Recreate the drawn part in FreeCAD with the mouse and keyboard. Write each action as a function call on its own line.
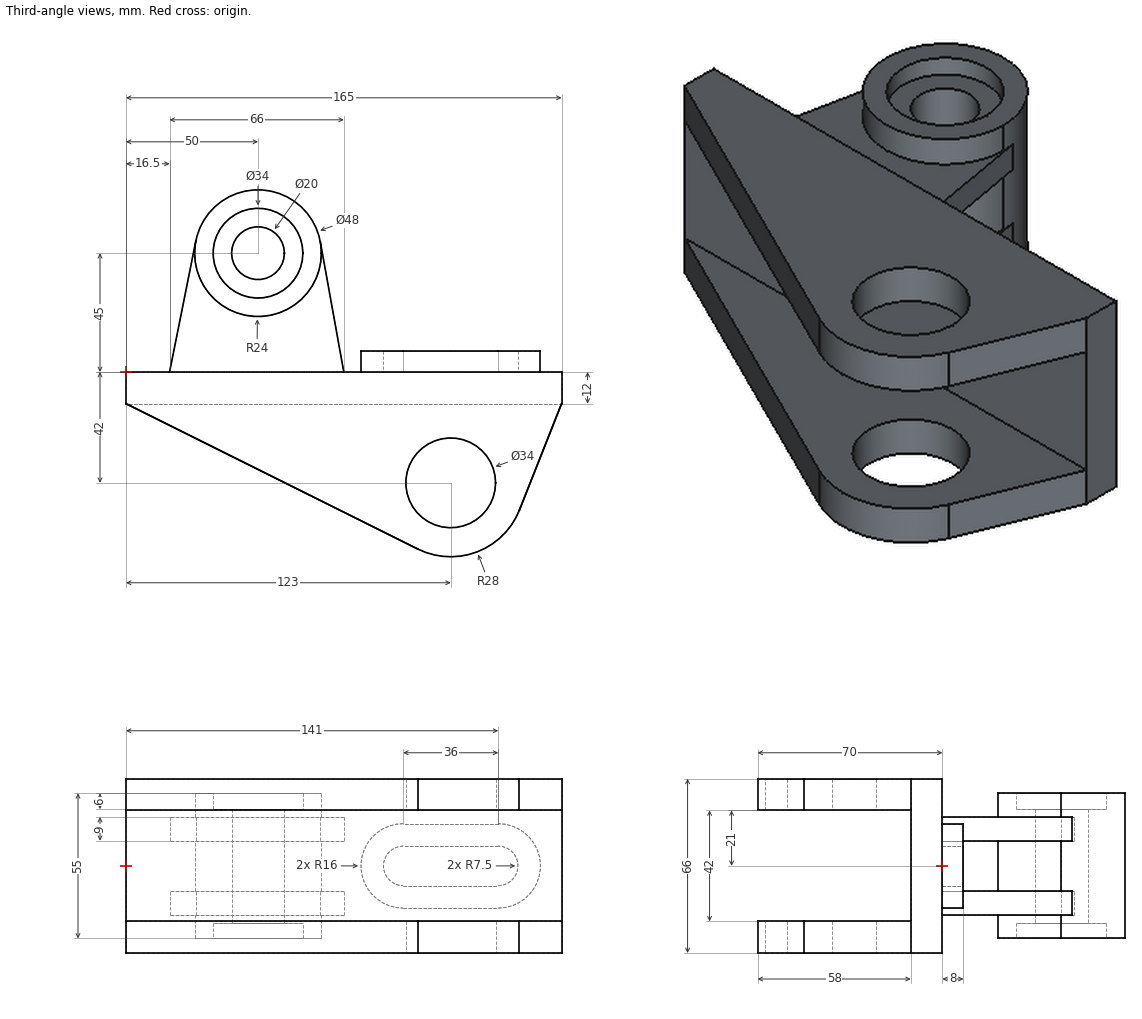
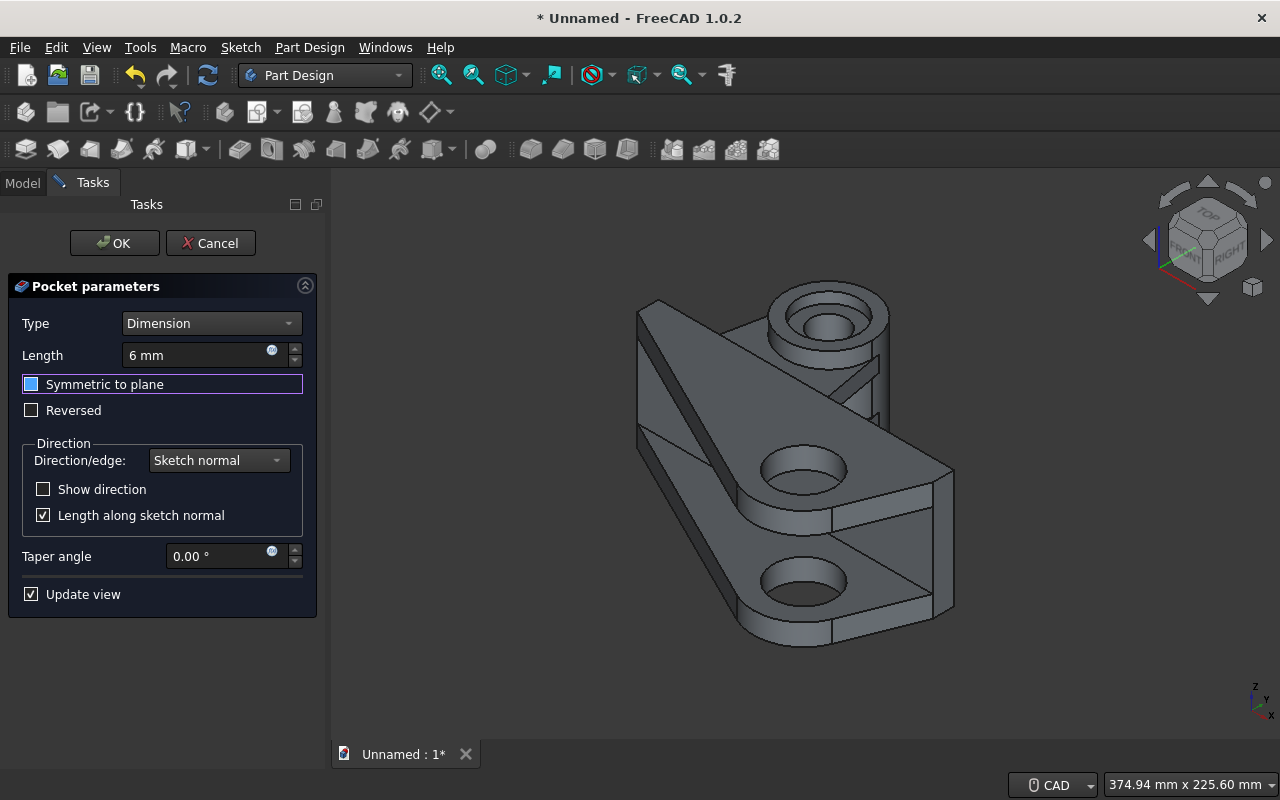
click(115, 243)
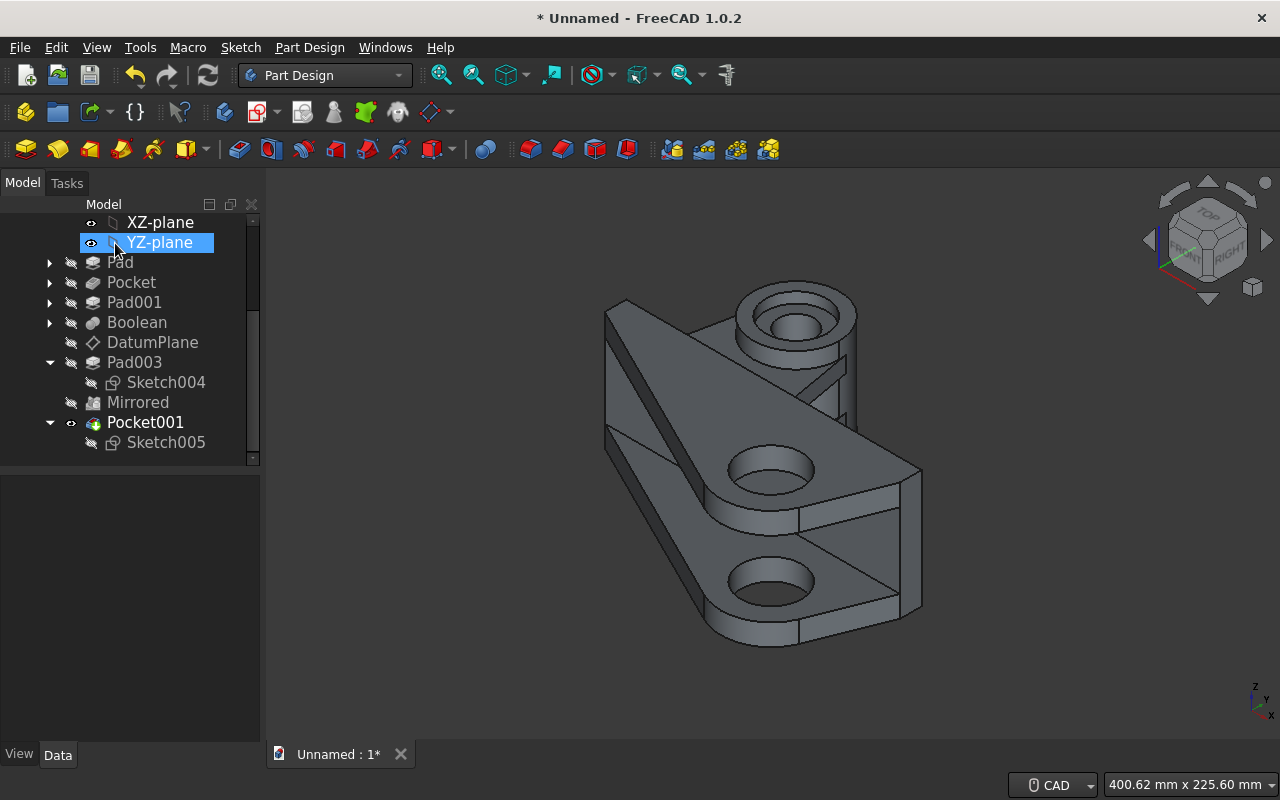
click(116, 423)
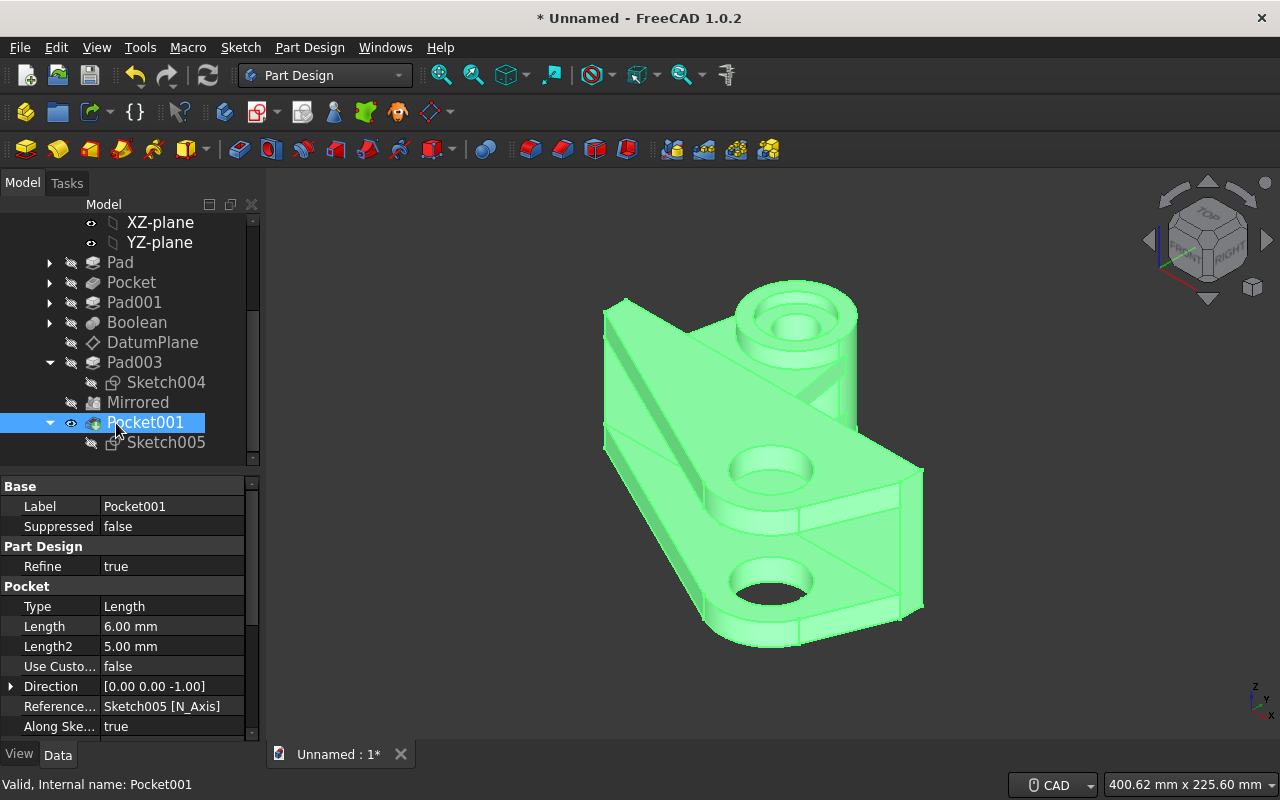
click(672, 150)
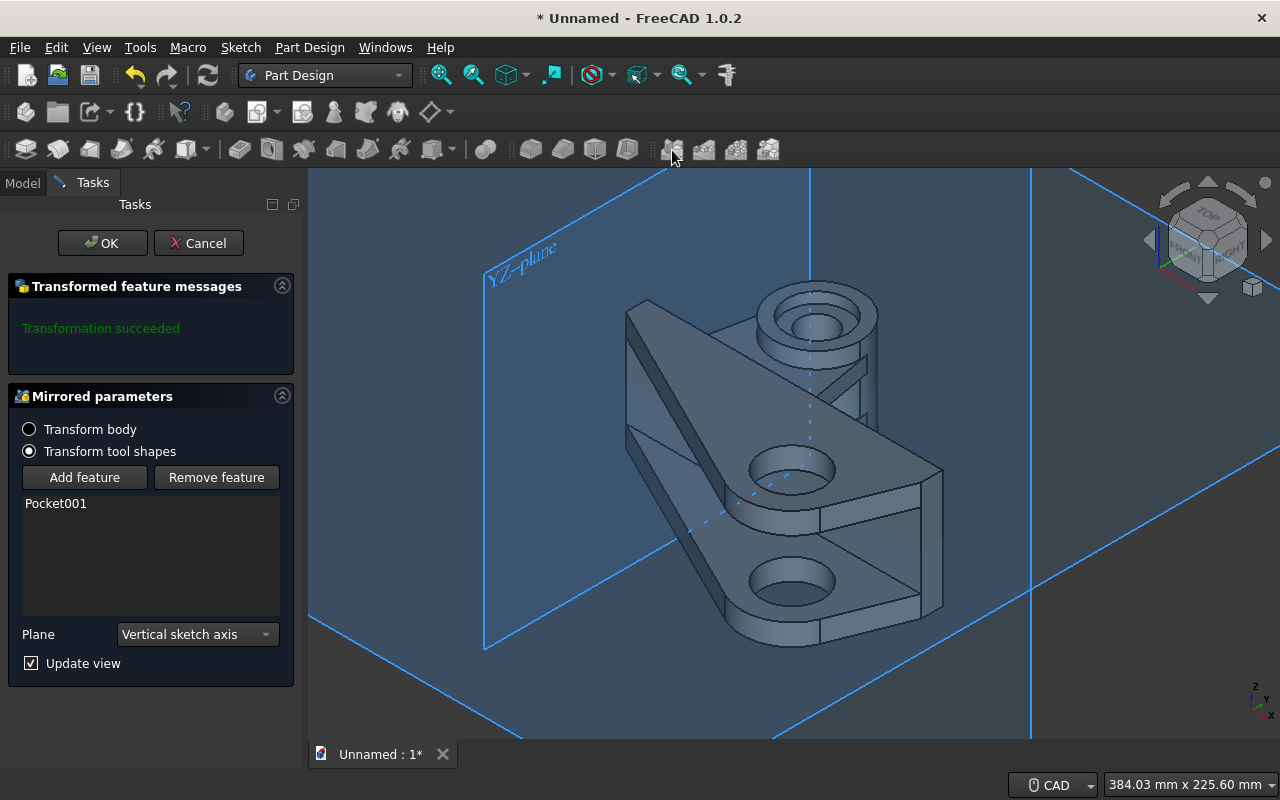
click(198, 634)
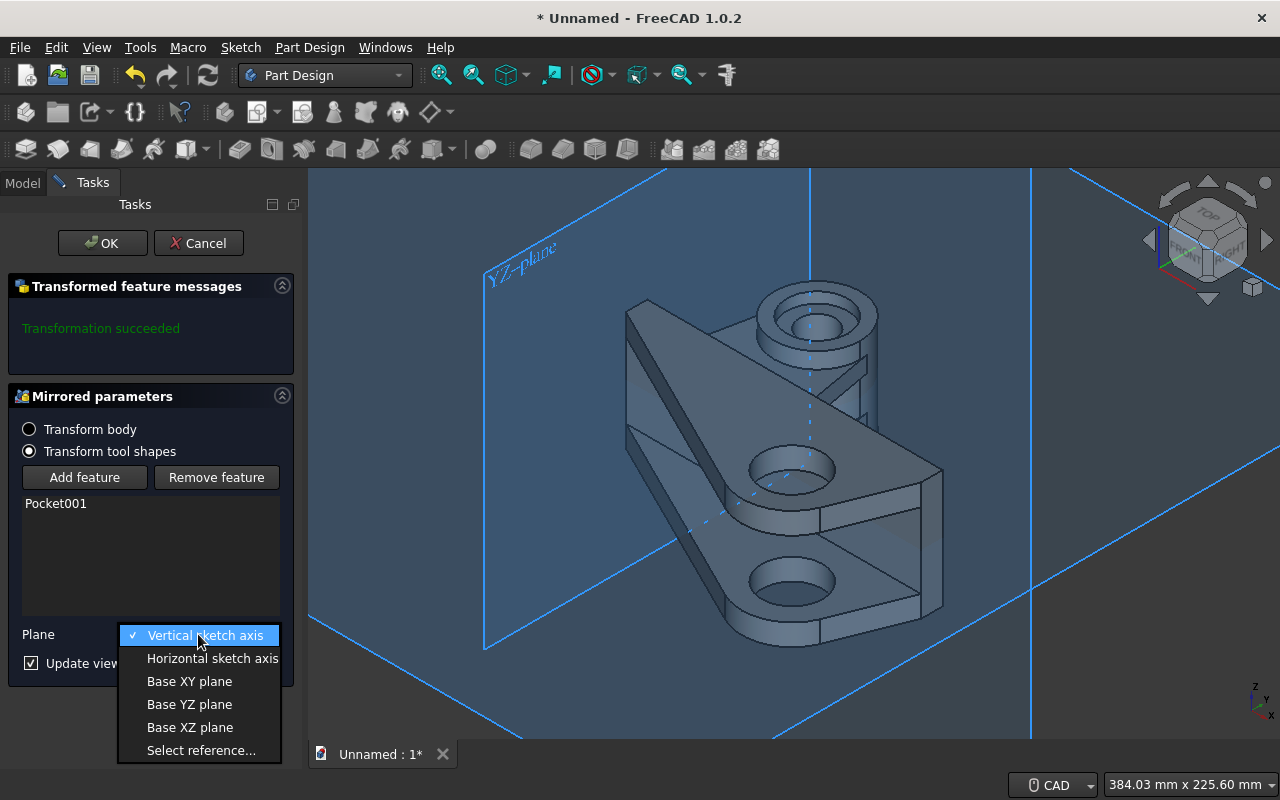
click(198, 682)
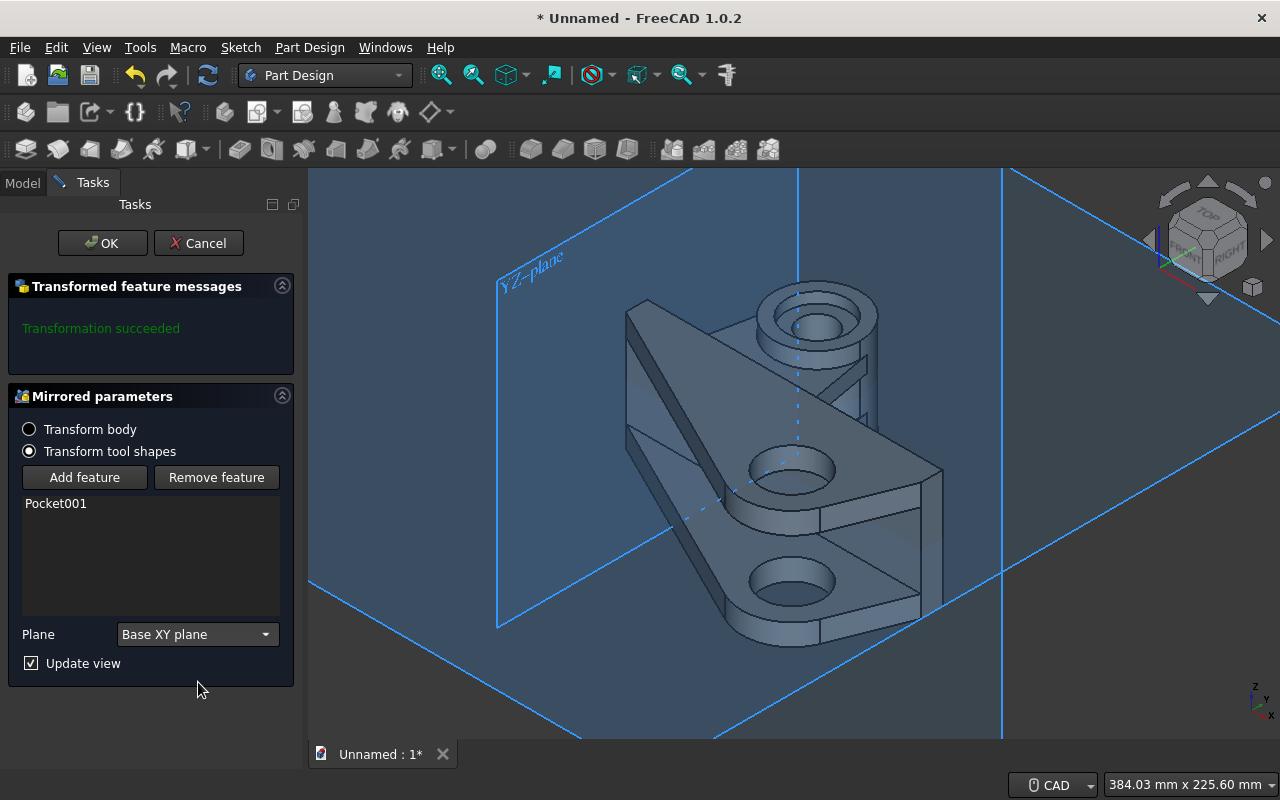
click(103, 243)